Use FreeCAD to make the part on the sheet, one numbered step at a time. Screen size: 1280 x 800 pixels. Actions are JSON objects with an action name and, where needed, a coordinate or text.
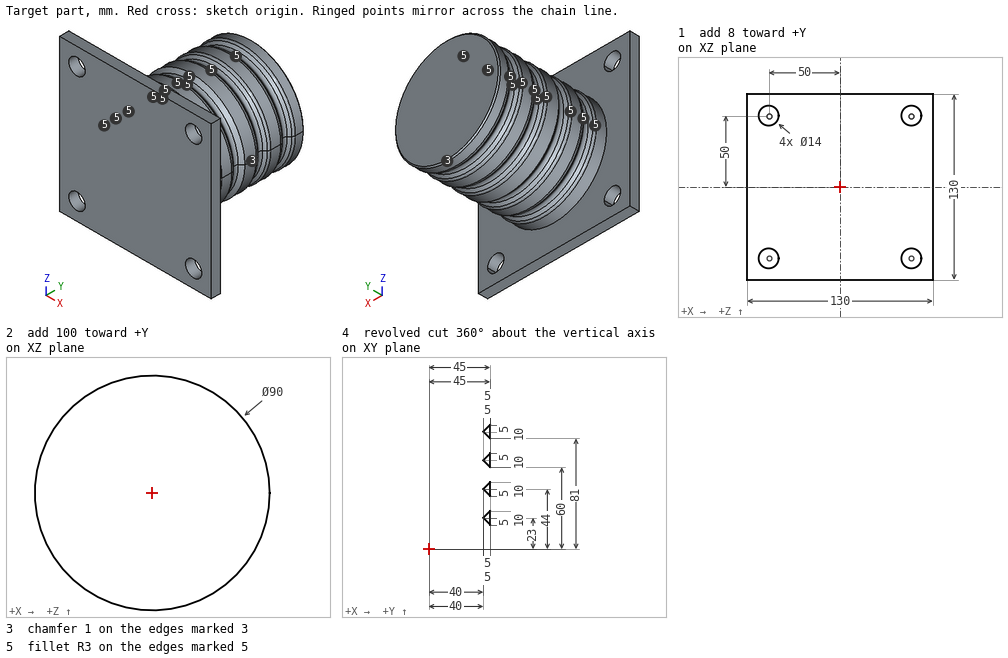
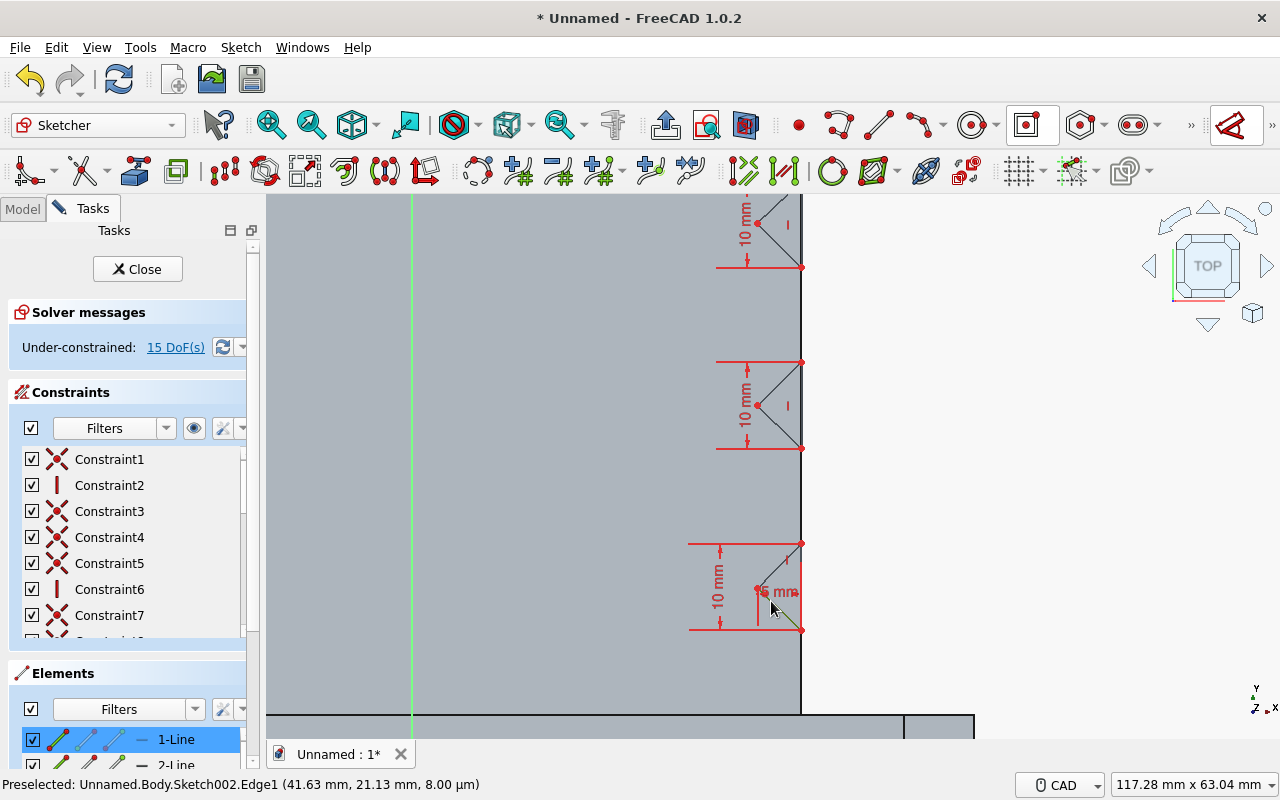
{"action": "left_click", "coordinate": [1258, 126]}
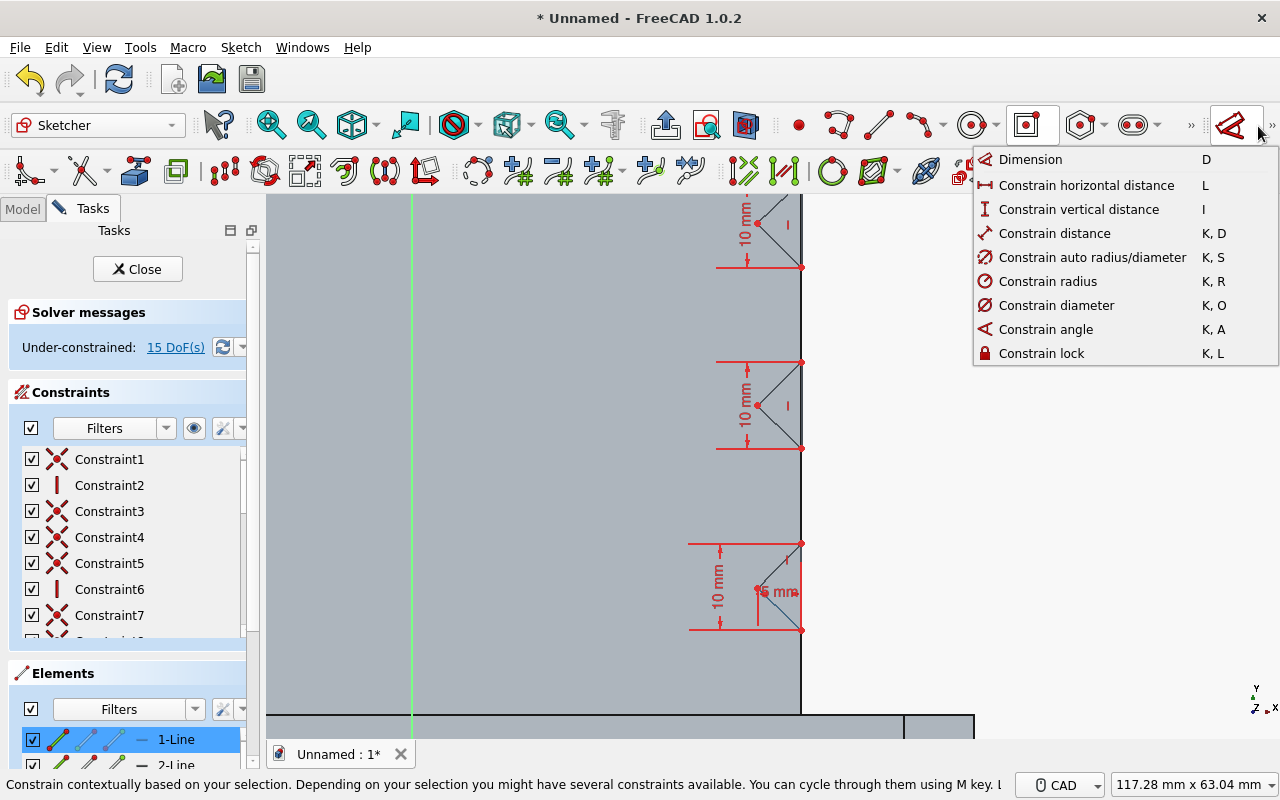
{"action": "left_click", "coordinate": [1126, 209]}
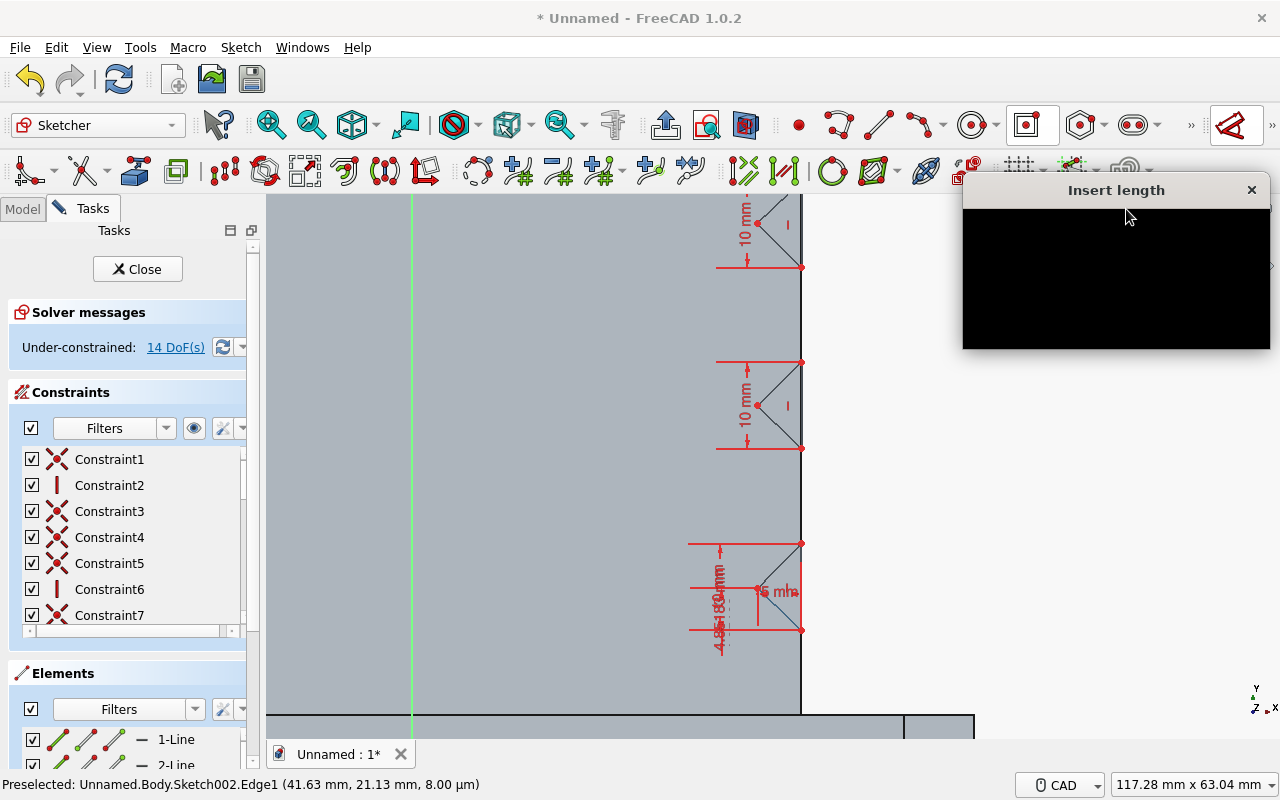
{"action": "type", "text": "5"}
{"action": "key", "text": "Return"}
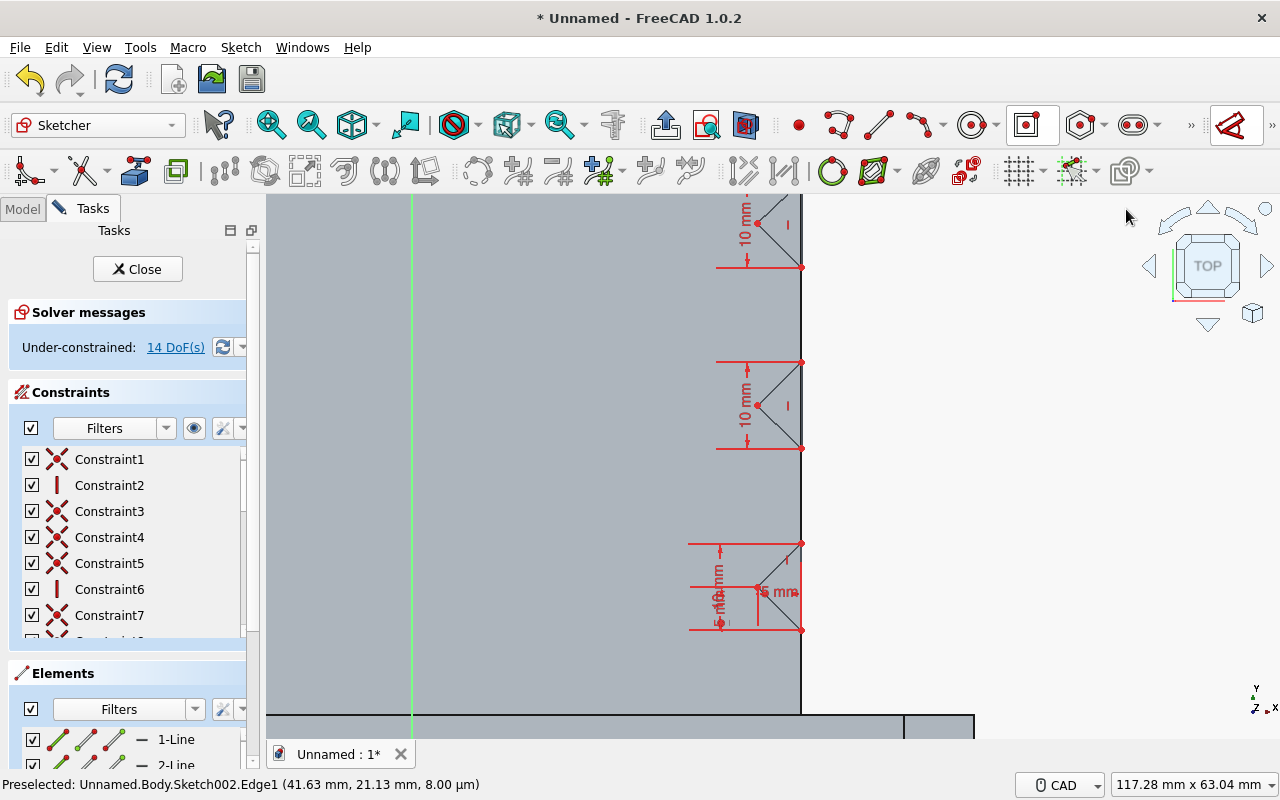
{"action": "left_click", "coordinate": [771, 419]}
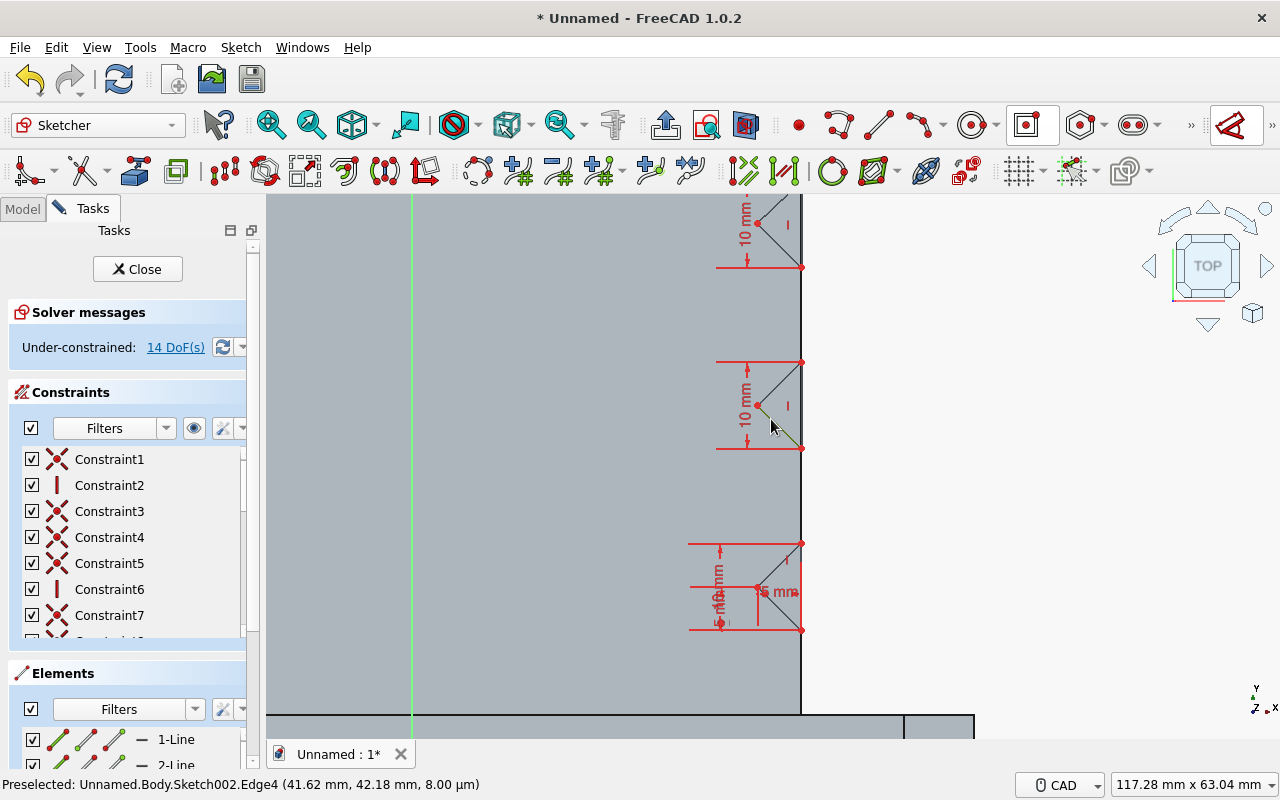
{"action": "key", "text": "l"}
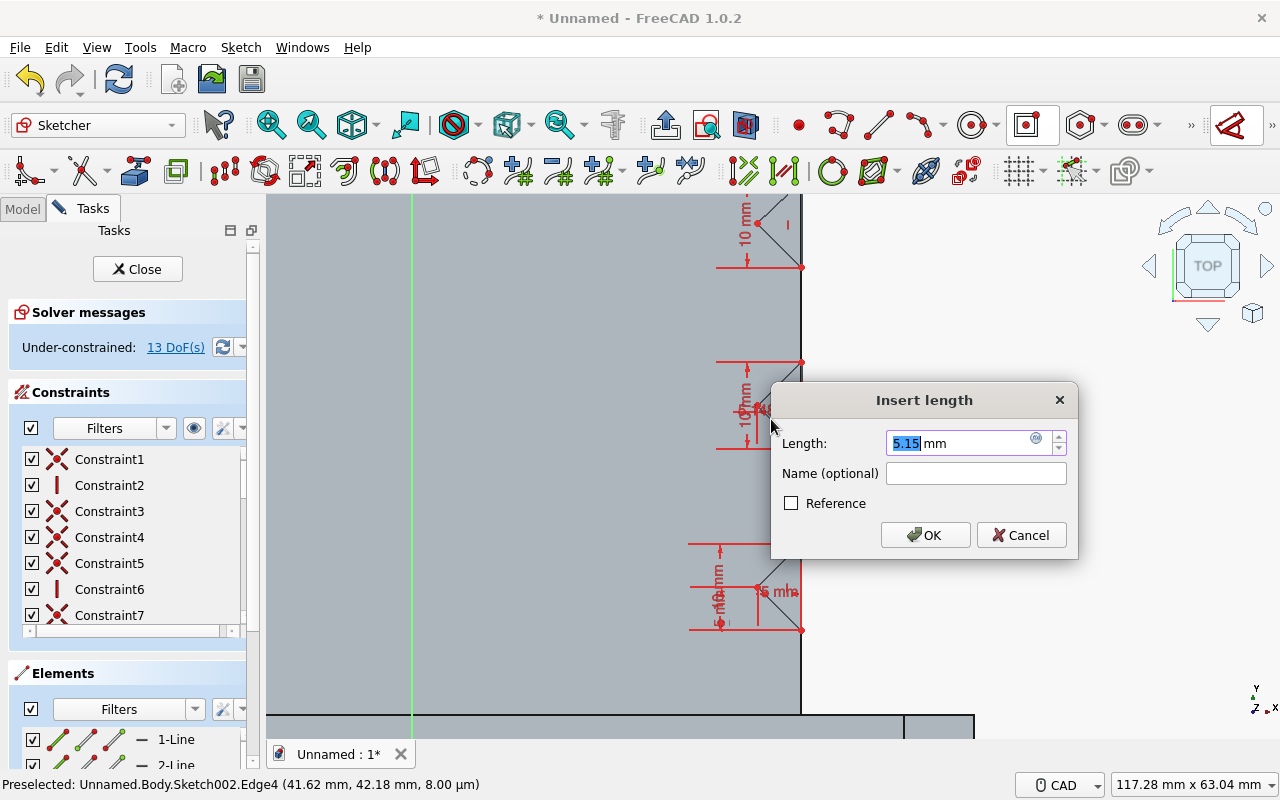
{"action": "type", "text": "5"}
{"action": "key", "text": "Return"}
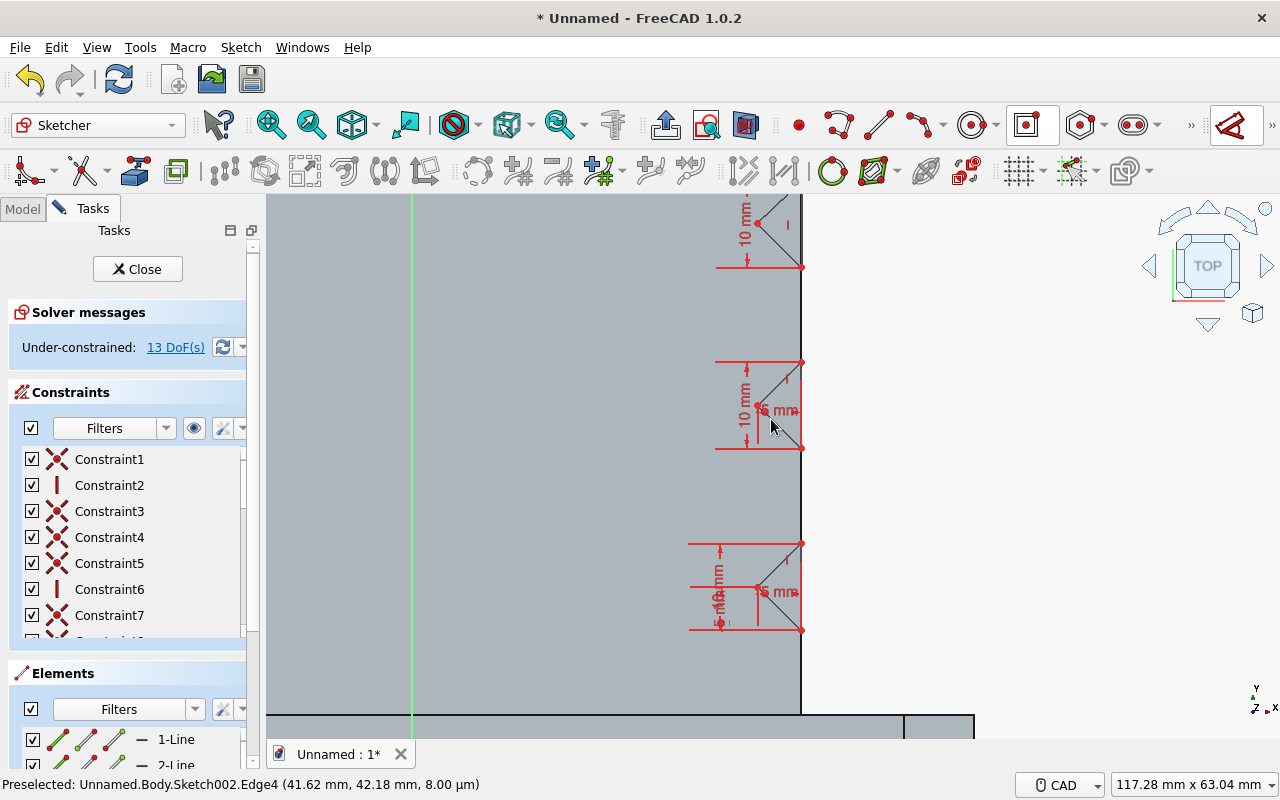
{"action": "left_click", "coordinate": [788, 436]}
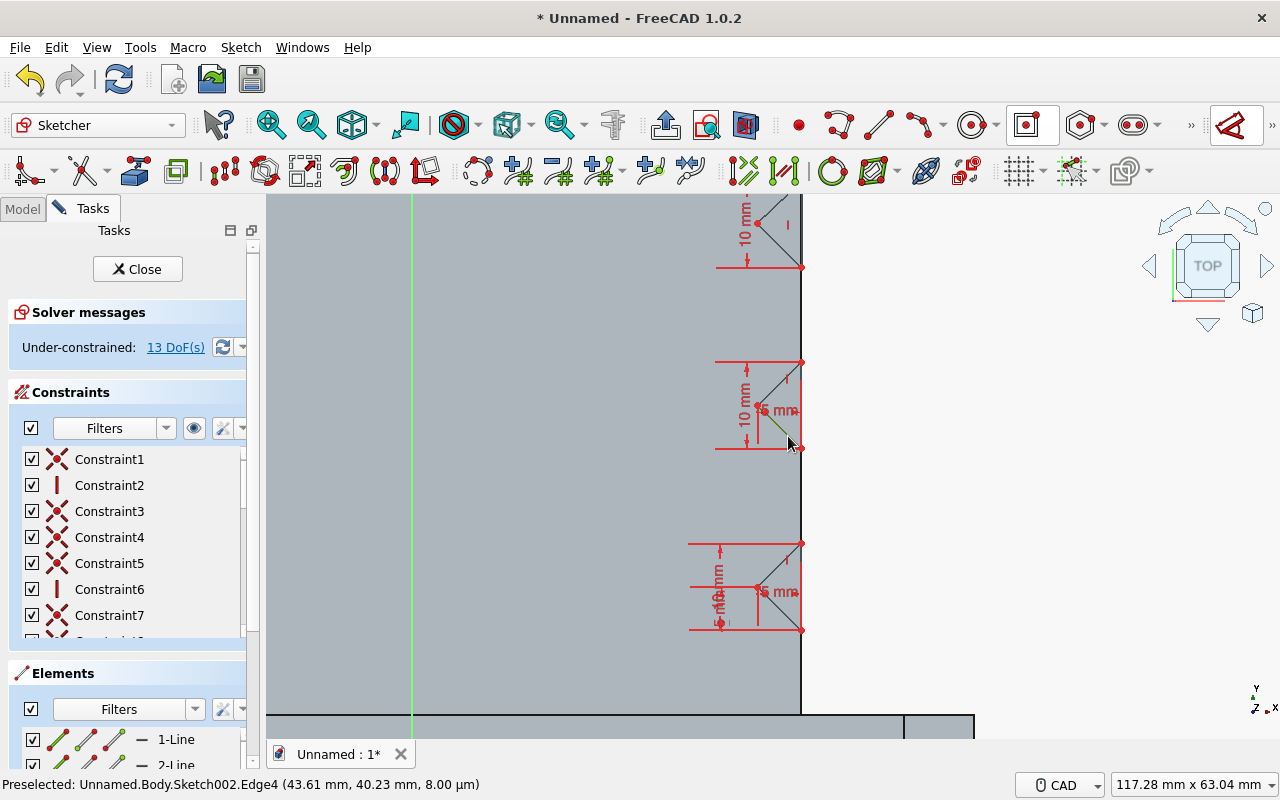
{"action": "key", "text": "i"}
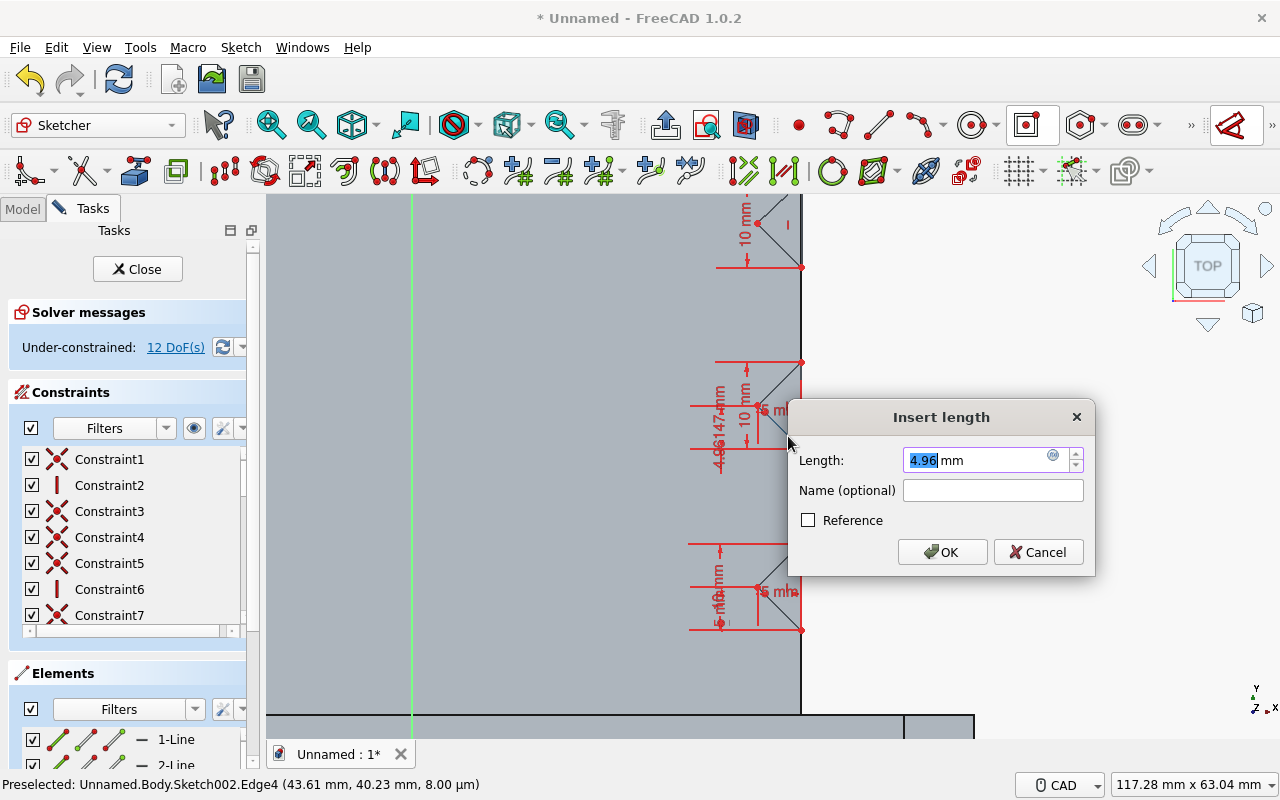
{"action": "type", "text": "5"}
{"action": "key", "text": "Return"}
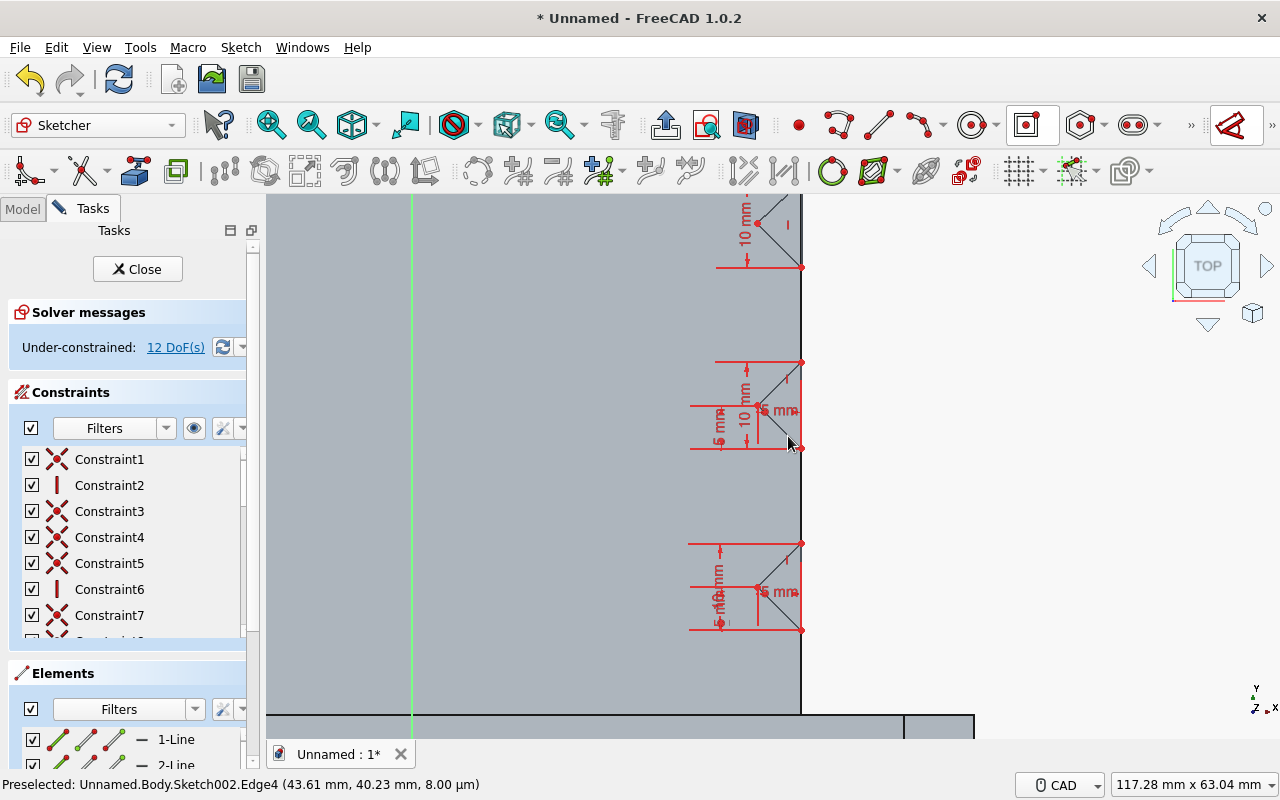
{"action": "scroll", "coordinate": [785, 528], "scroll_direction": "down", "scroll_amount": 4}